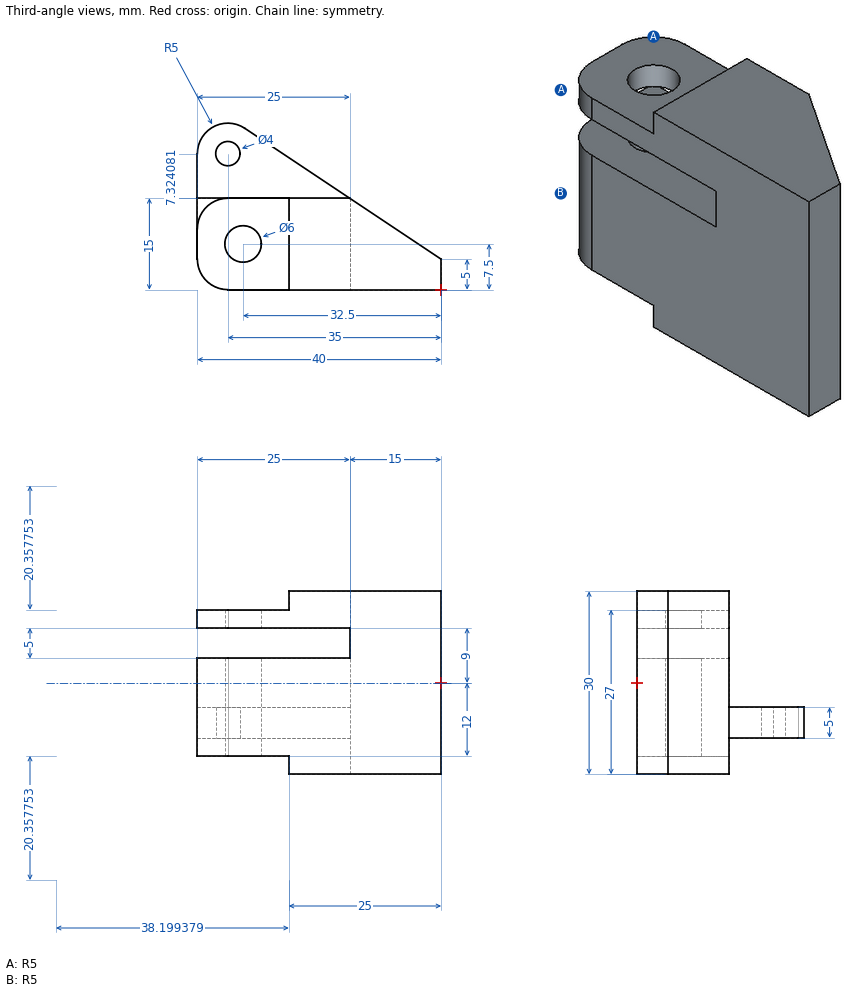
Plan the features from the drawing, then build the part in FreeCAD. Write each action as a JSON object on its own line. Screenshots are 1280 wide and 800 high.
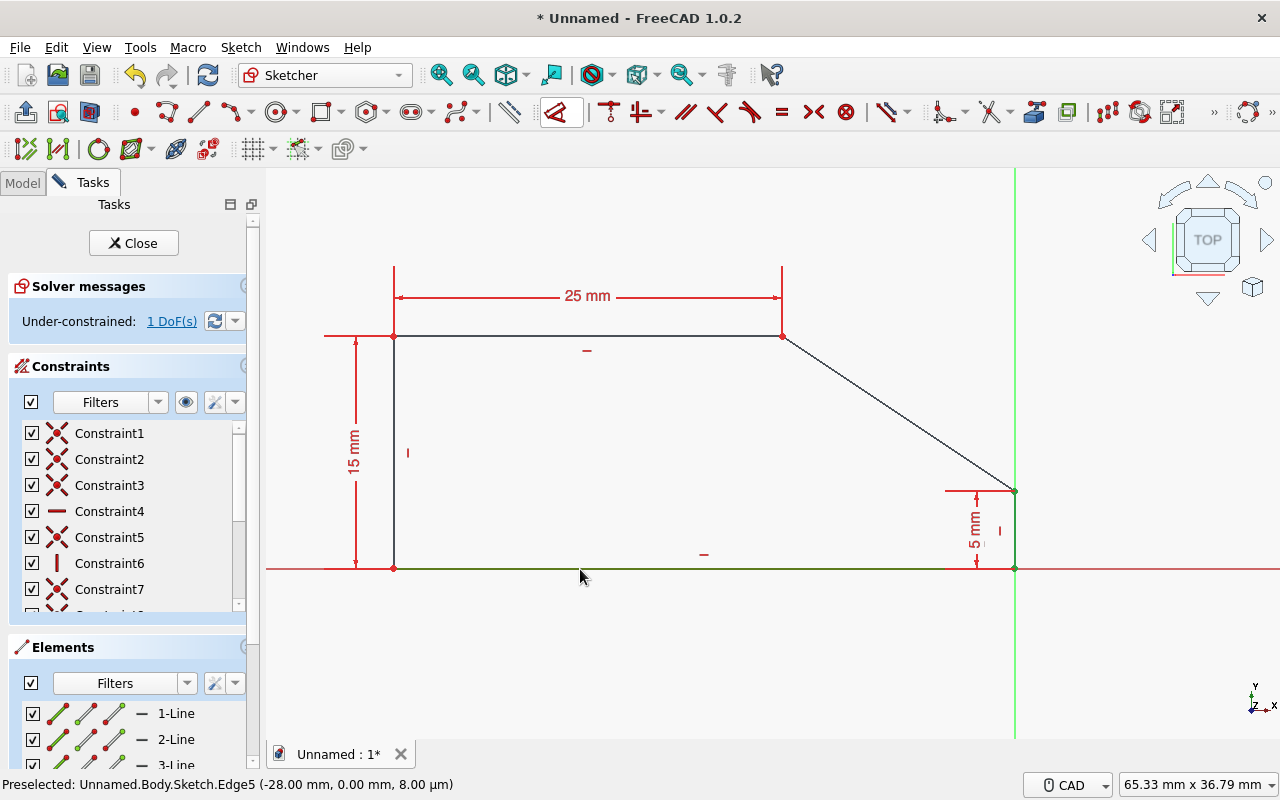
{"action": "left_click", "coordinate": [578, 112]}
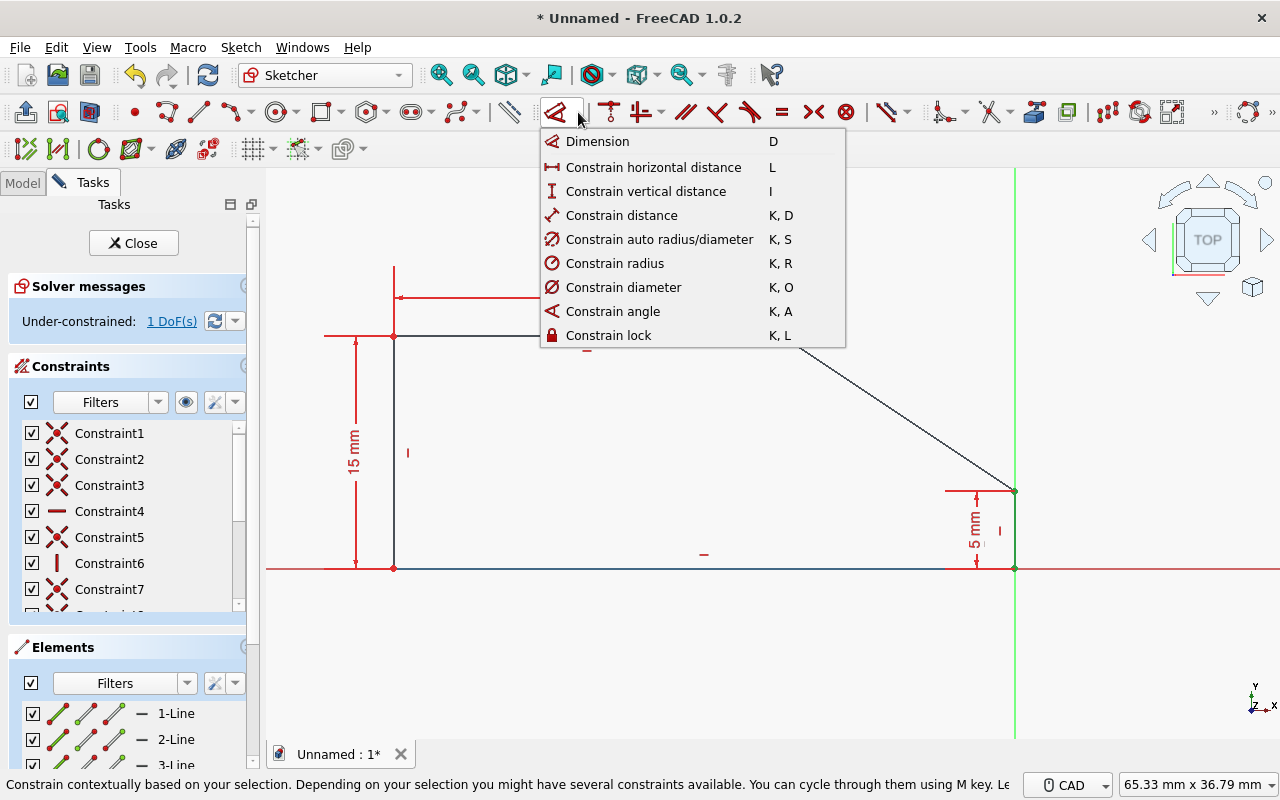
{"action": "left_click", "coordinate": [693, 167]}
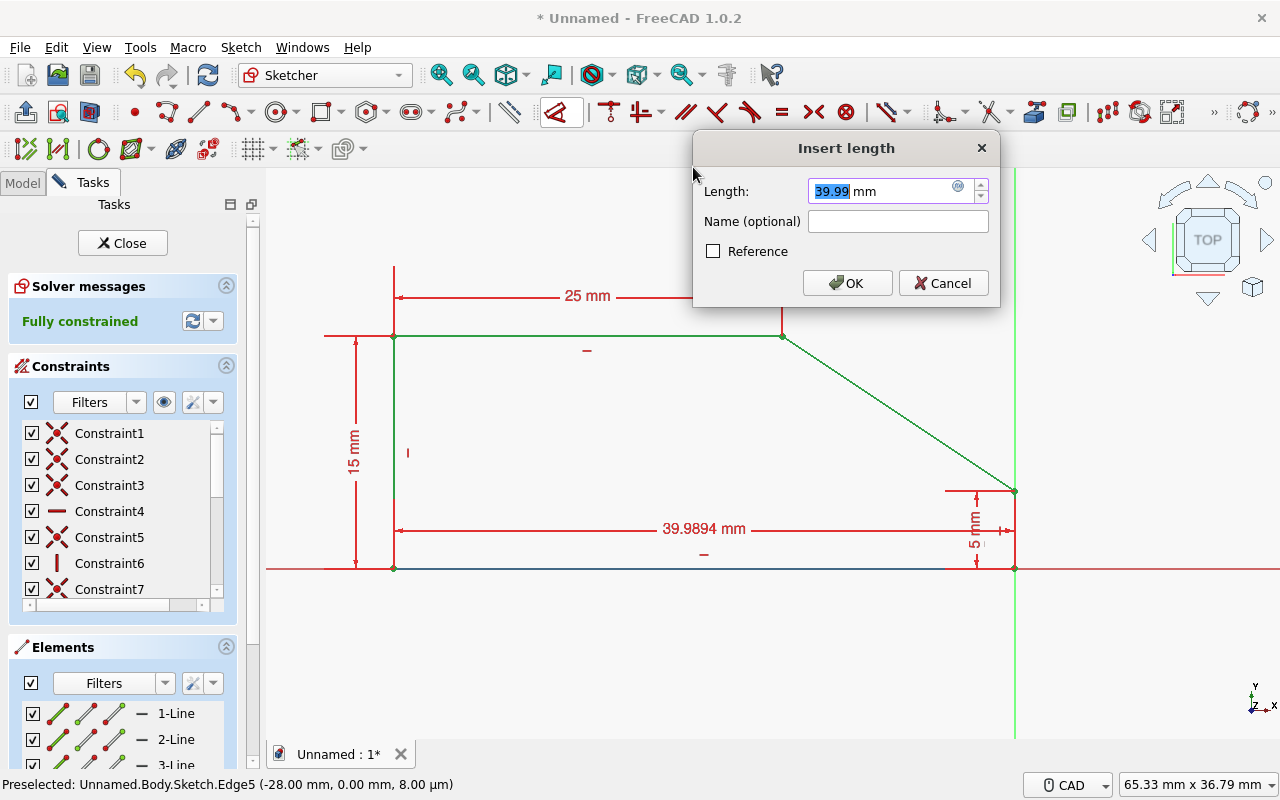
{"action": "type", "text": "40"}
{"action": "key", "text": "Return"}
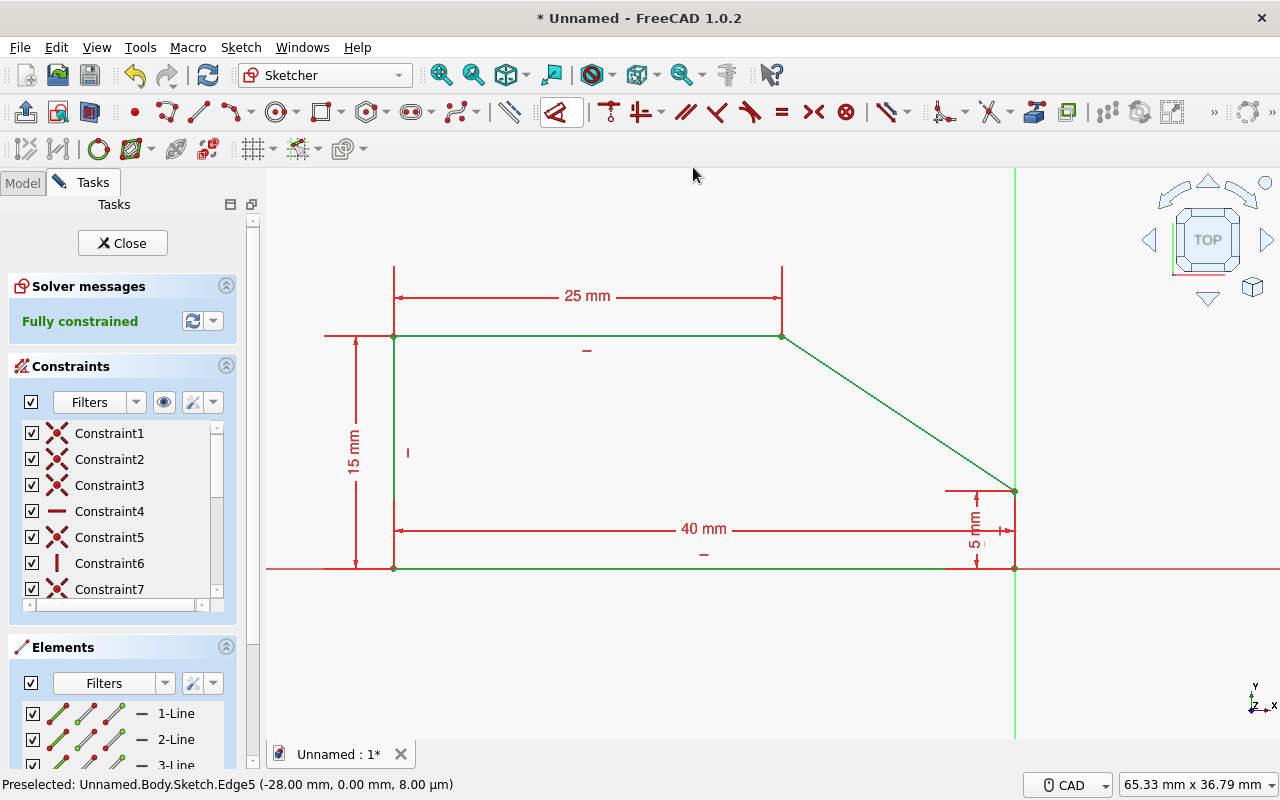
{"action": "left_click", "coordinate": [123, 243]}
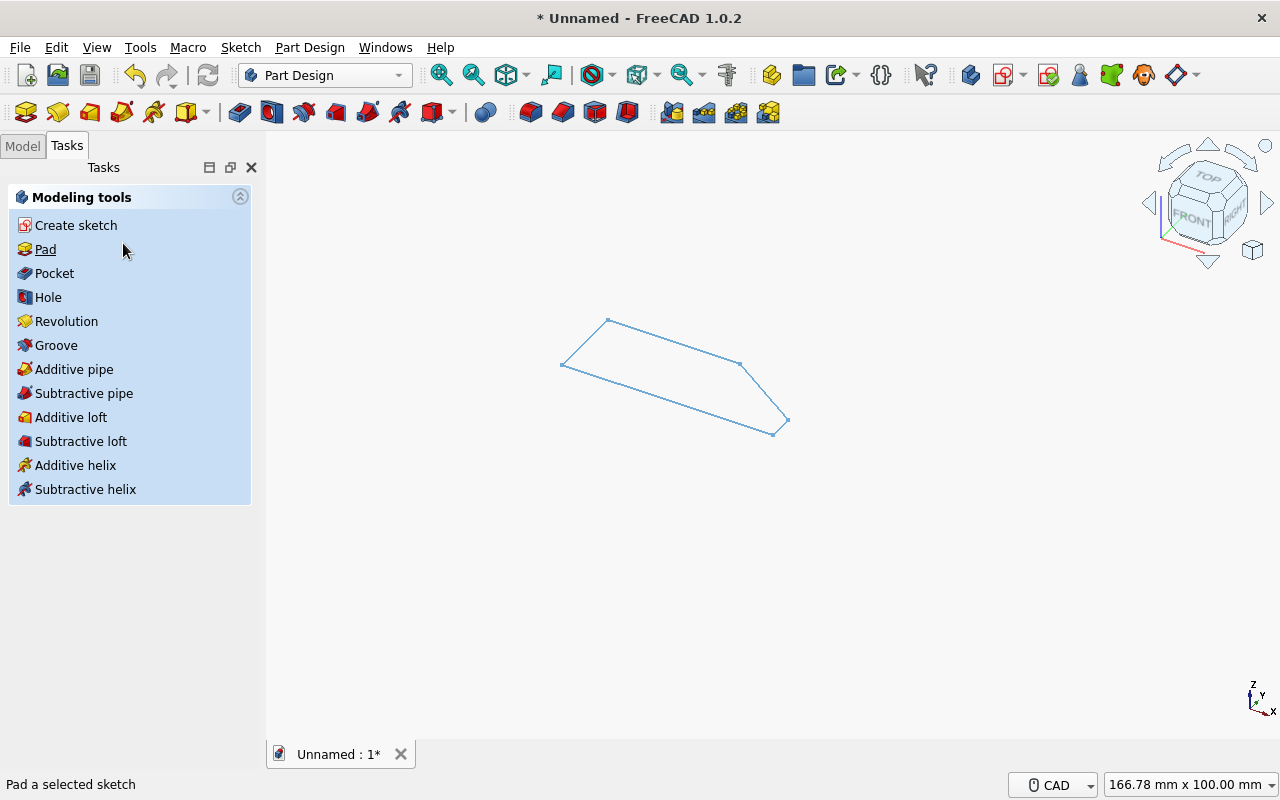
{"action": "left_click", "coordinate": [26, 112]}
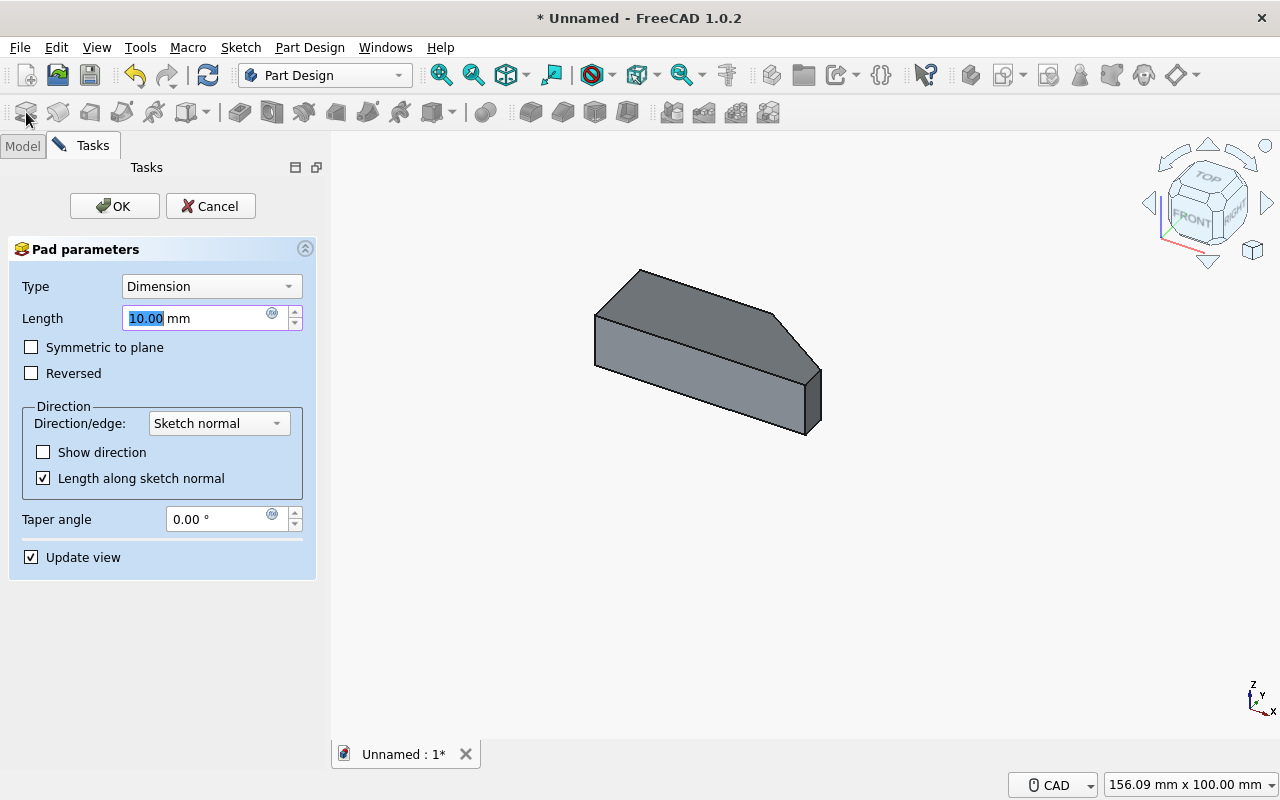
{"action": "type", "text": "30"}
{"action": "key", "text": "Tab"}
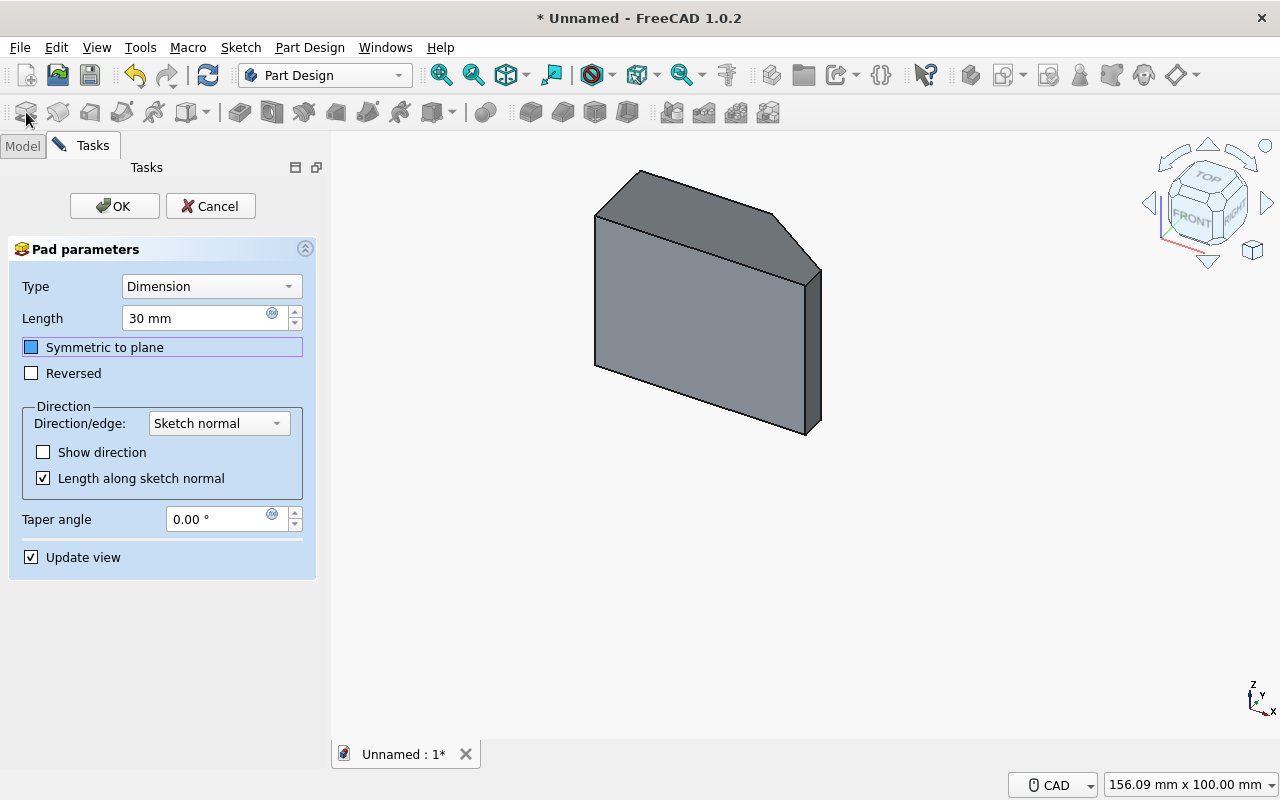
{"action": "left_click", "coordinate": [30, 347]}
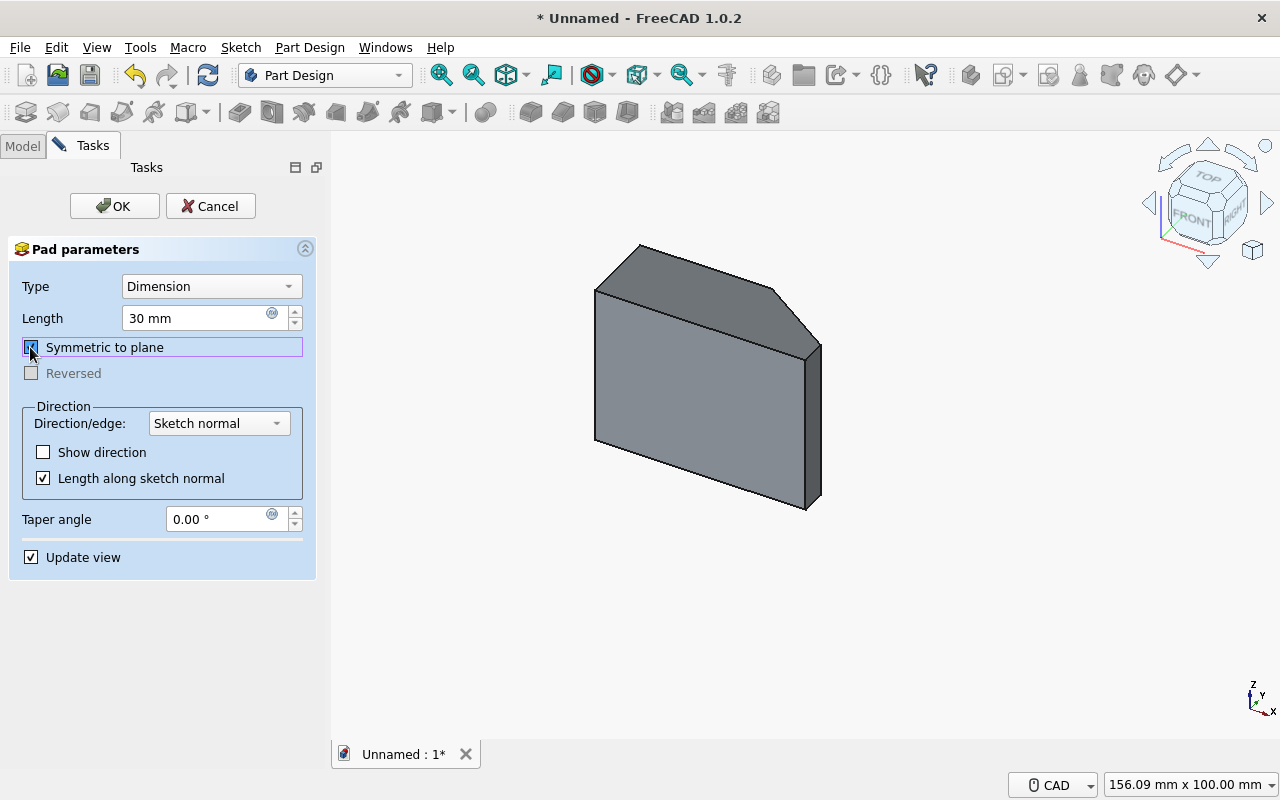
{"action": "left_click", "coordinate": [115, 206]}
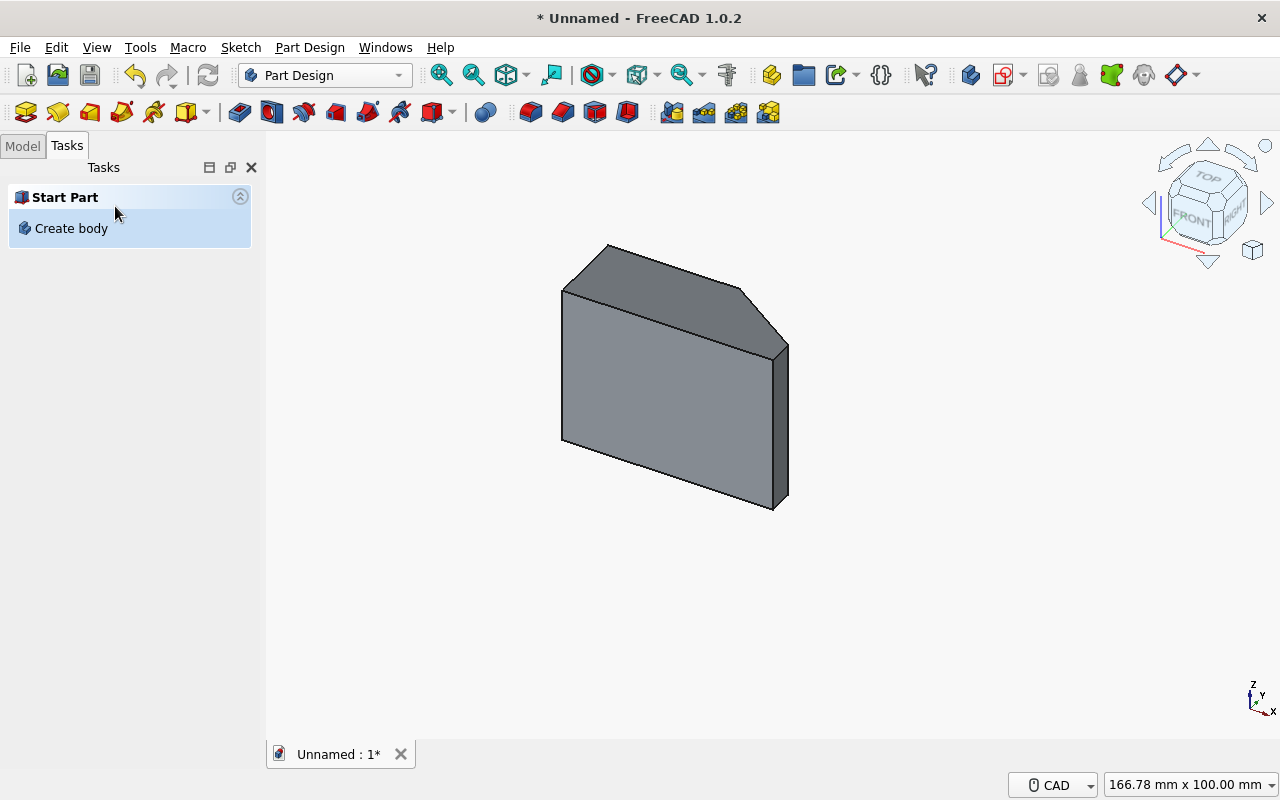
{"action": "key", "text": "v f"}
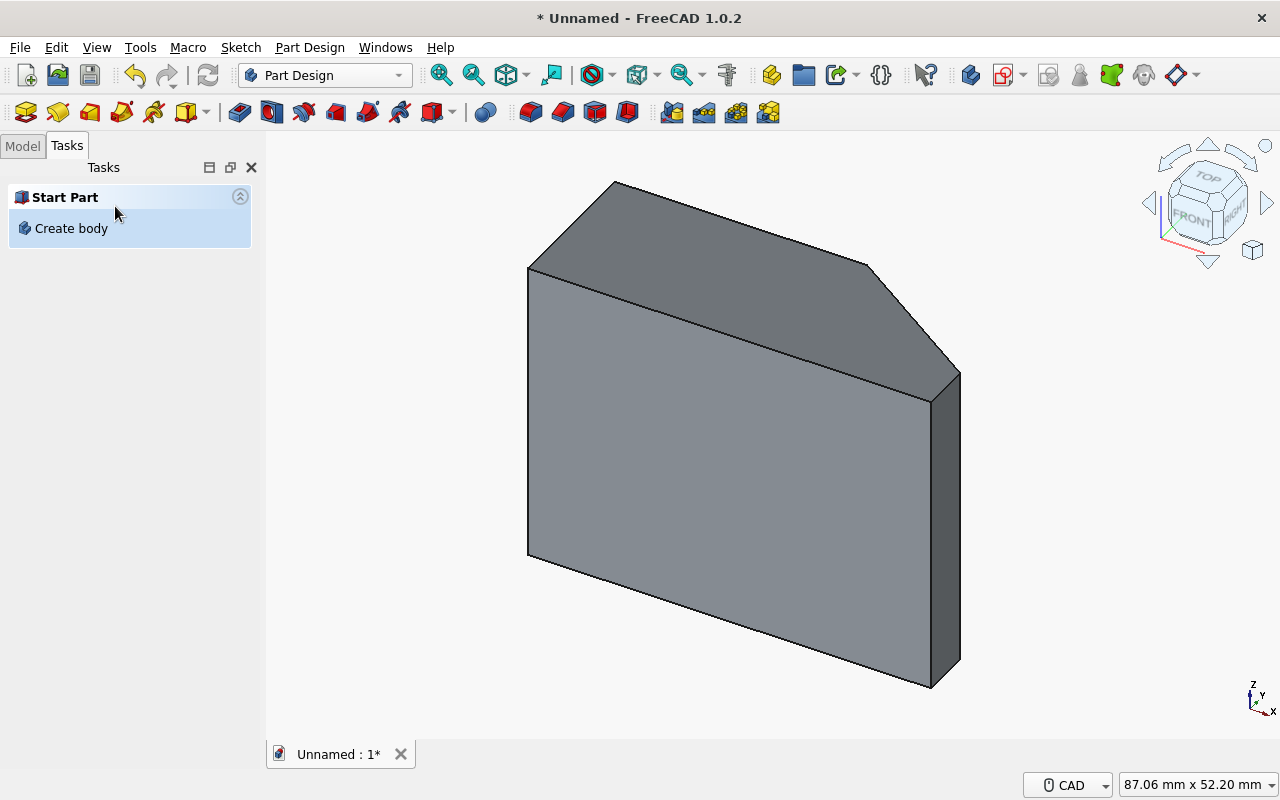
{"action": "key", "text": "4"}